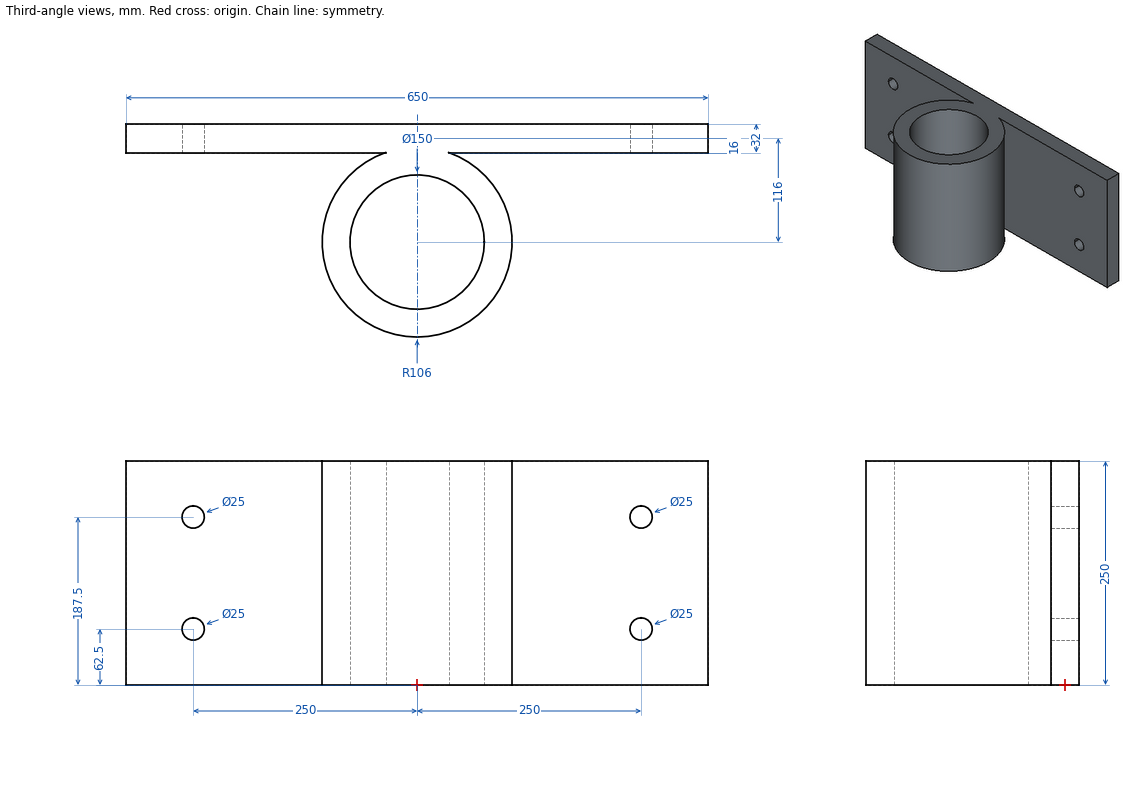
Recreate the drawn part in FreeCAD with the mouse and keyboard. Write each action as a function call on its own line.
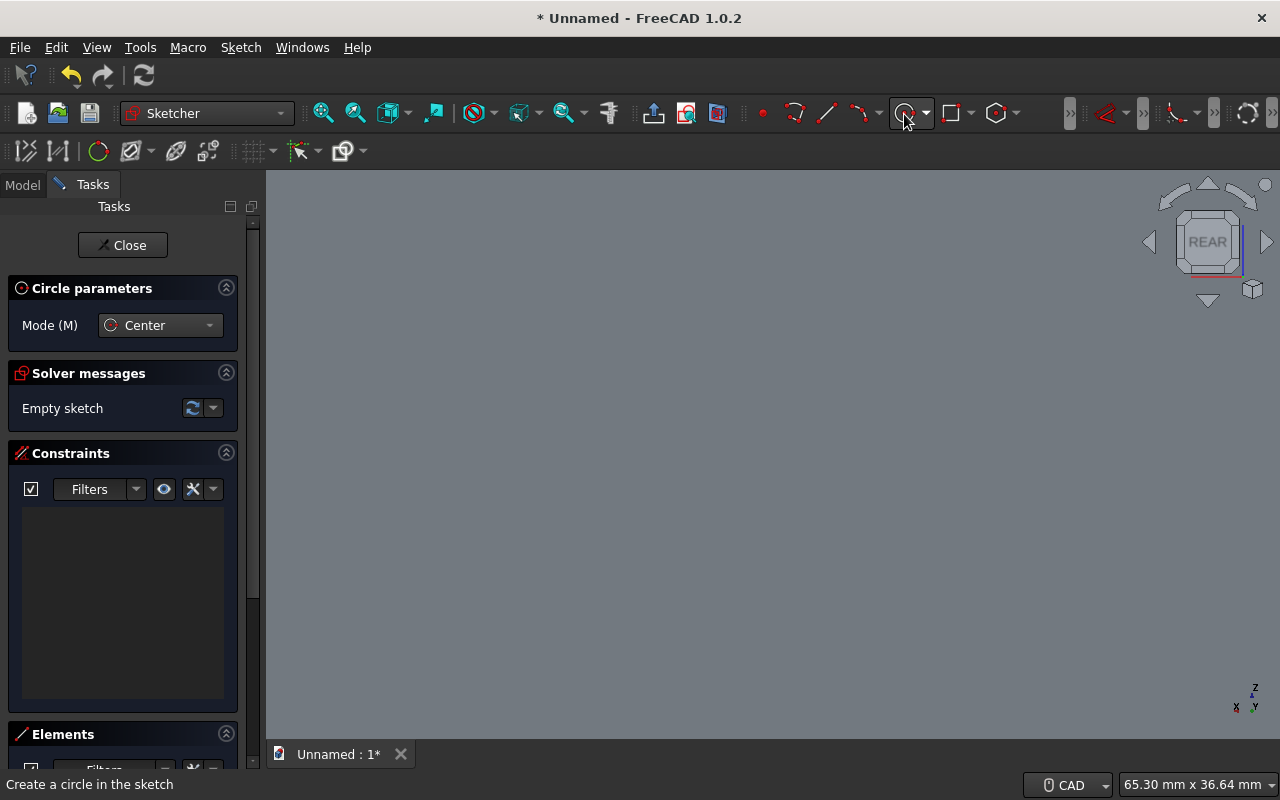
click(702, 450)
click(839, 313)
key(Escape)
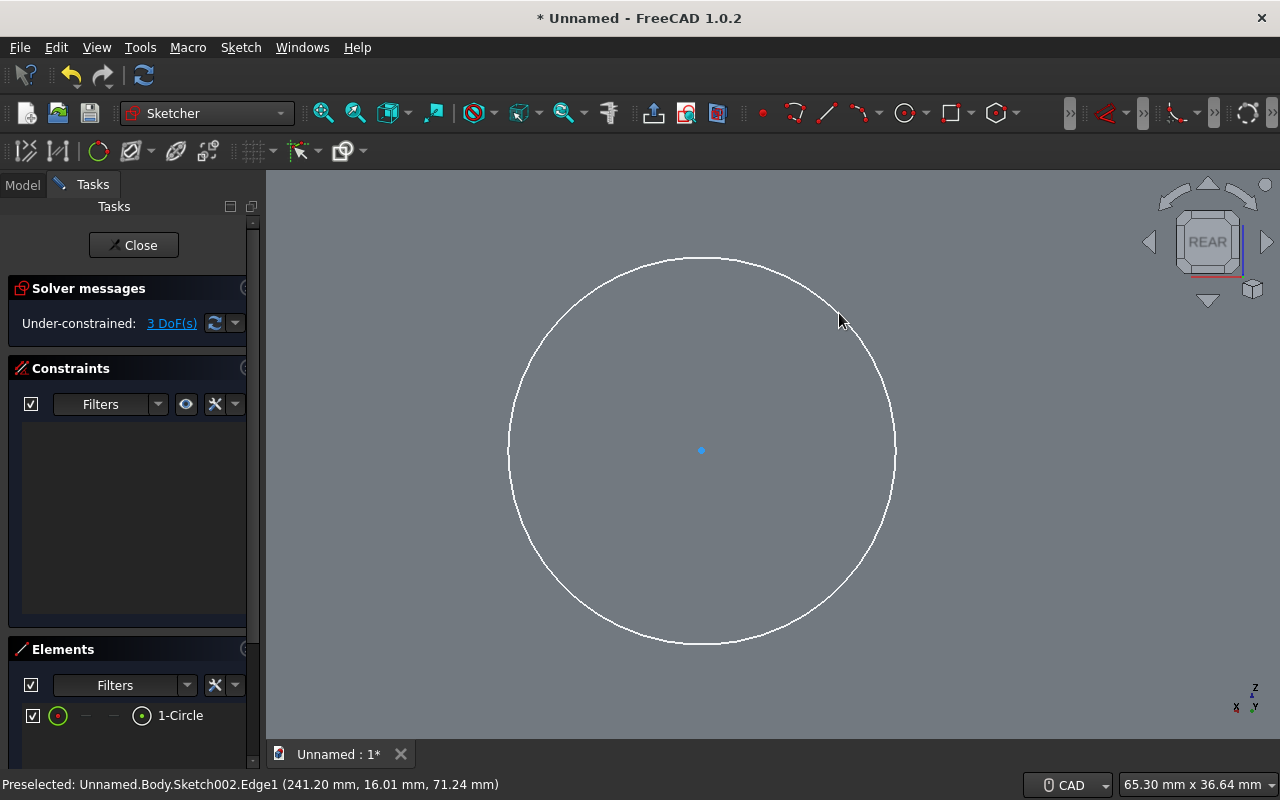
click(1106, 114)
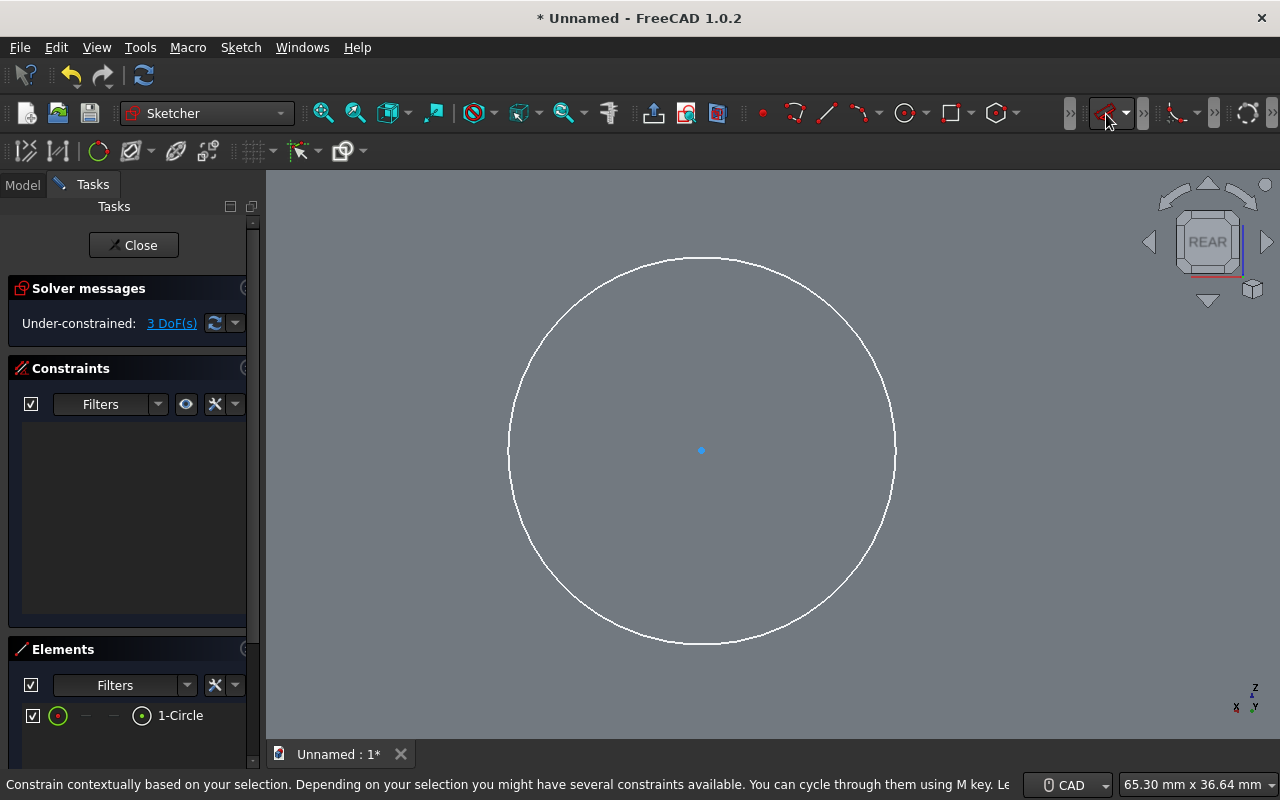
click(839, 314)
click(862, 291)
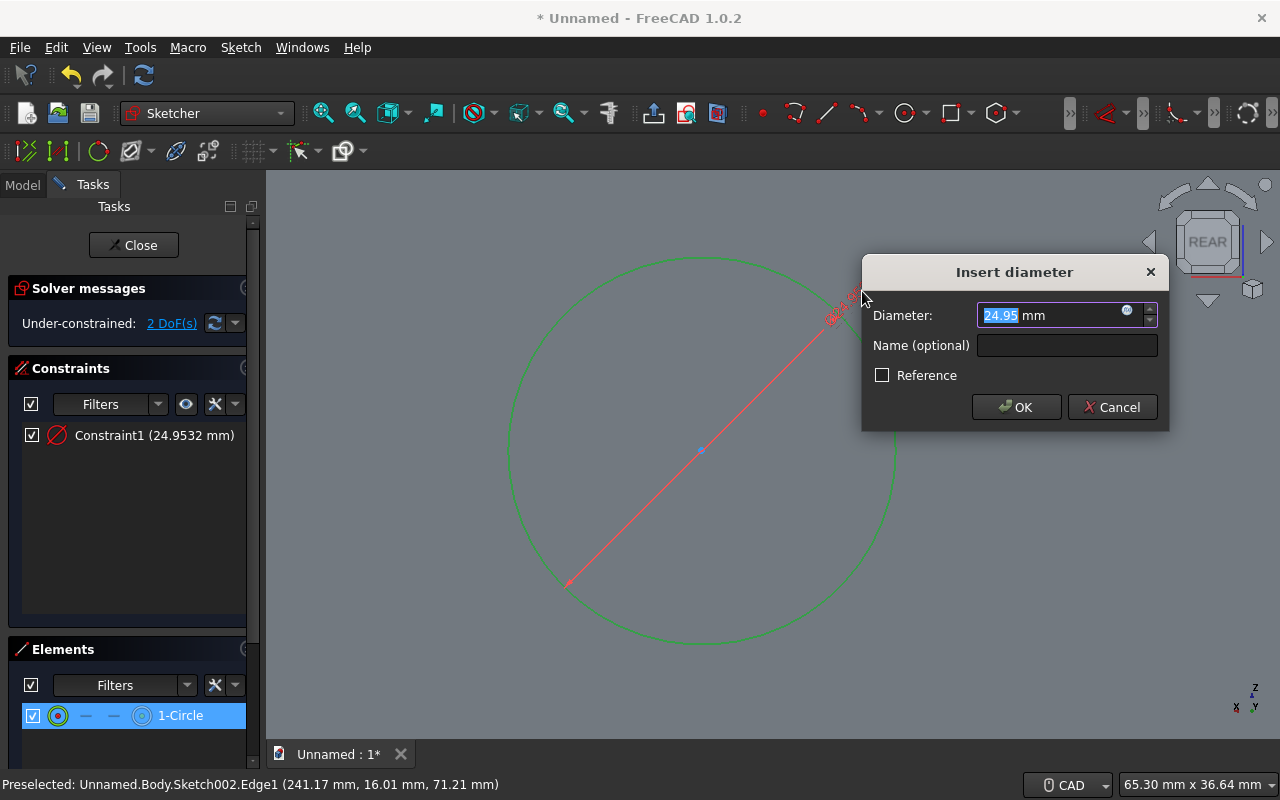
text(25)
key(Return)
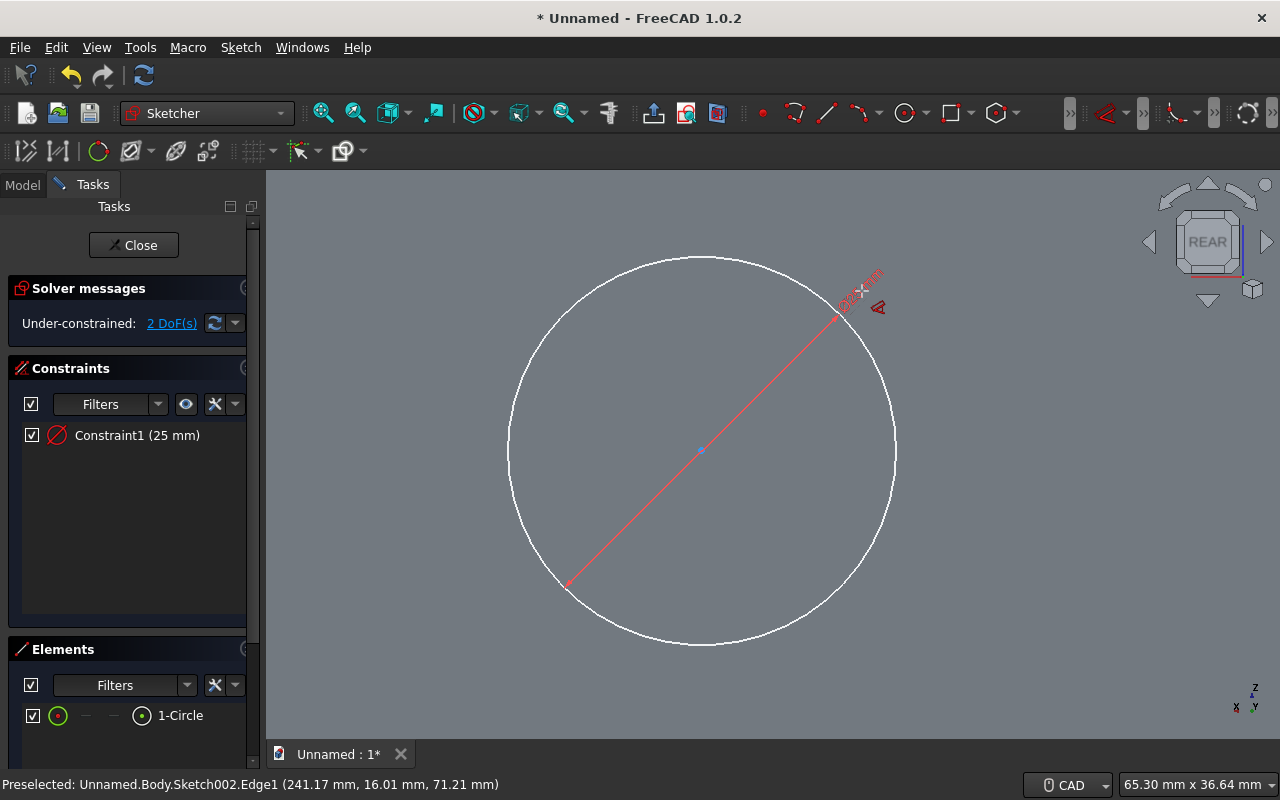
click(702, 451)
click(908, 417)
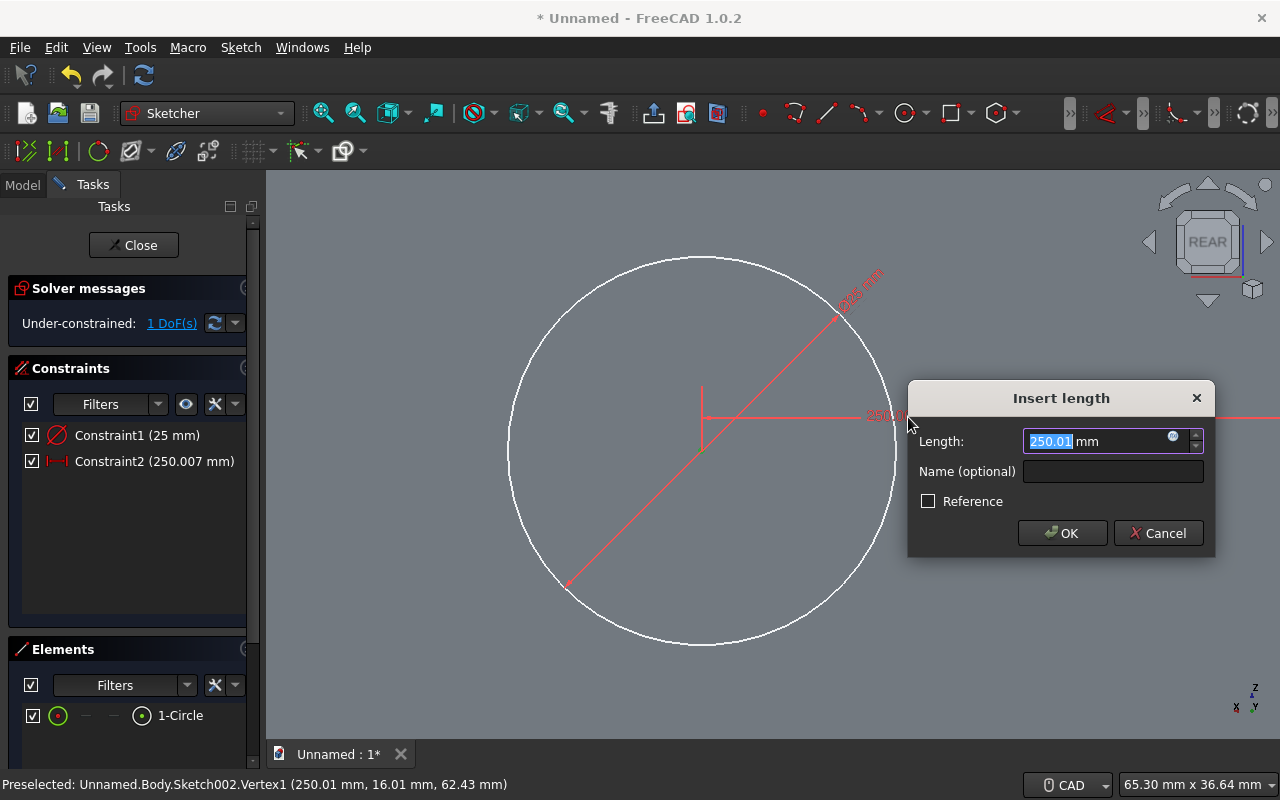
text(250)
key(Return)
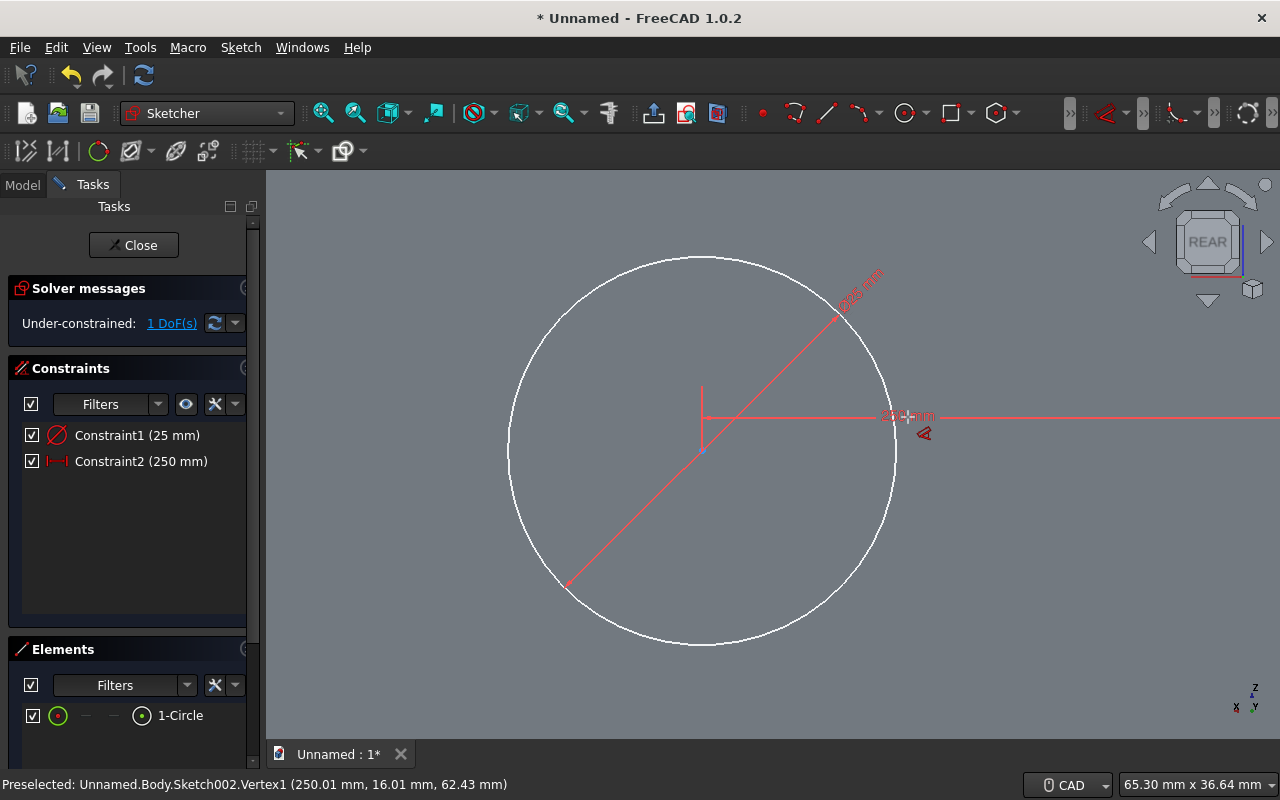
click(702, 451)
click(668, 581)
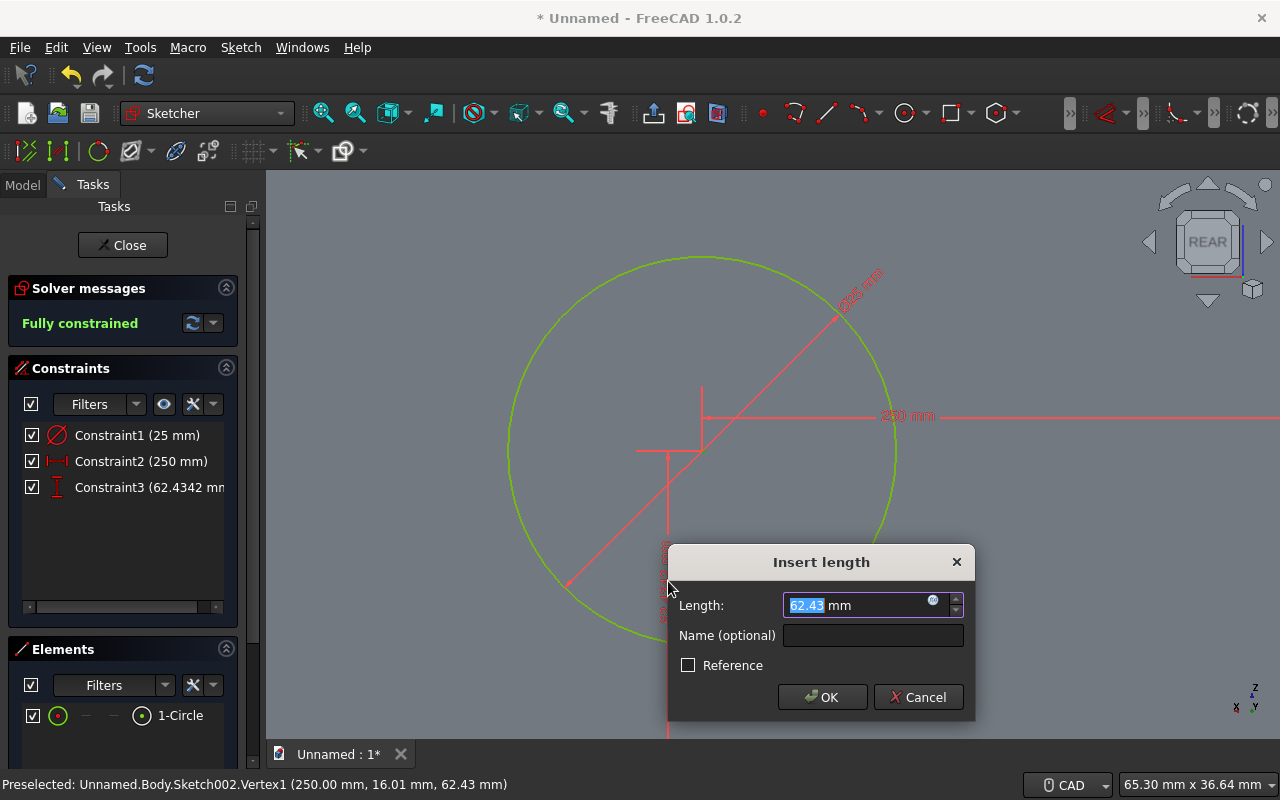
text(62.5)
key(Return)
key(Escape)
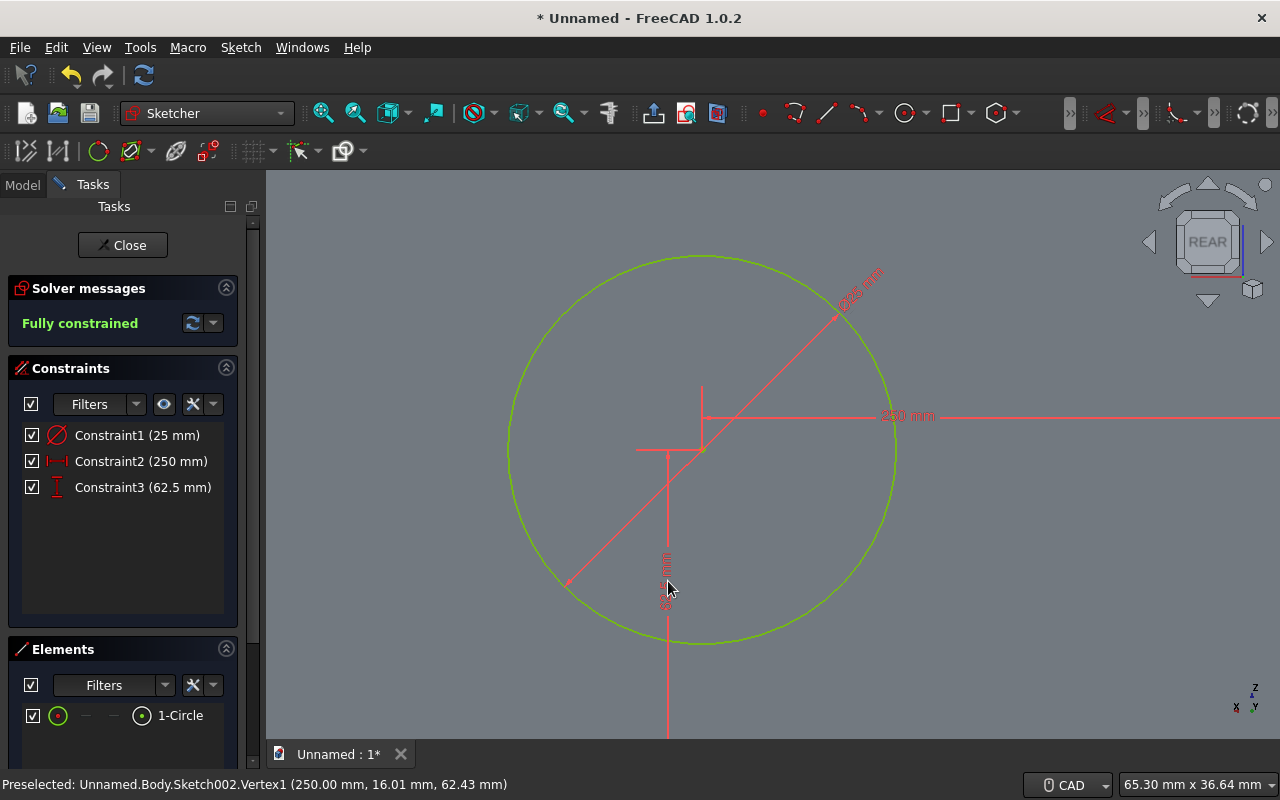
click(123, 245)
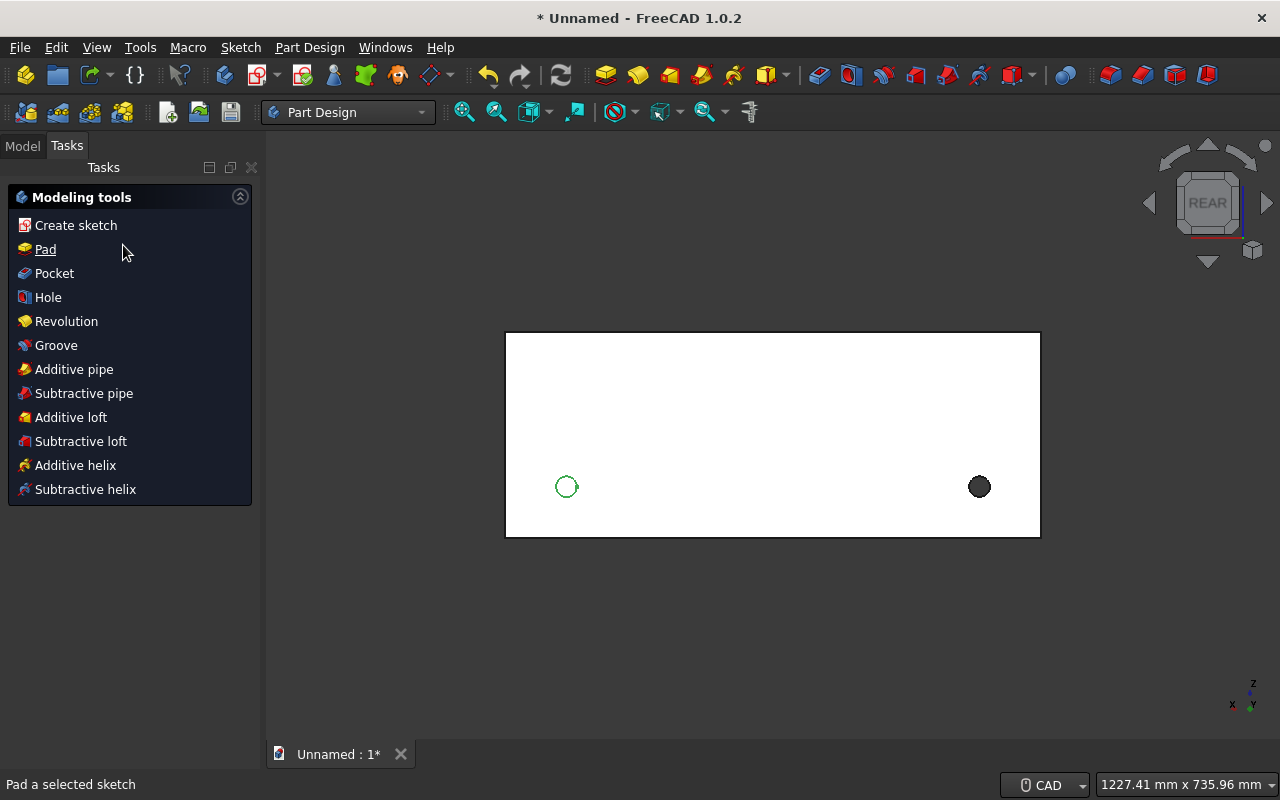
click(820, 76)